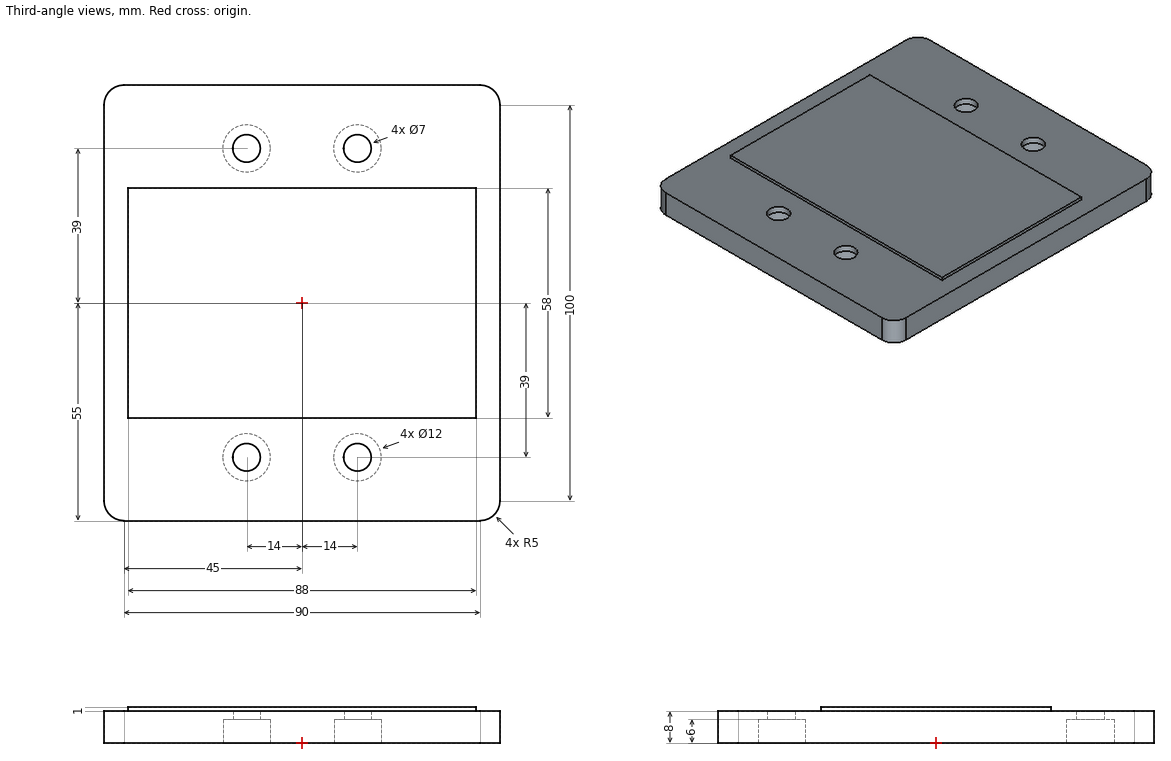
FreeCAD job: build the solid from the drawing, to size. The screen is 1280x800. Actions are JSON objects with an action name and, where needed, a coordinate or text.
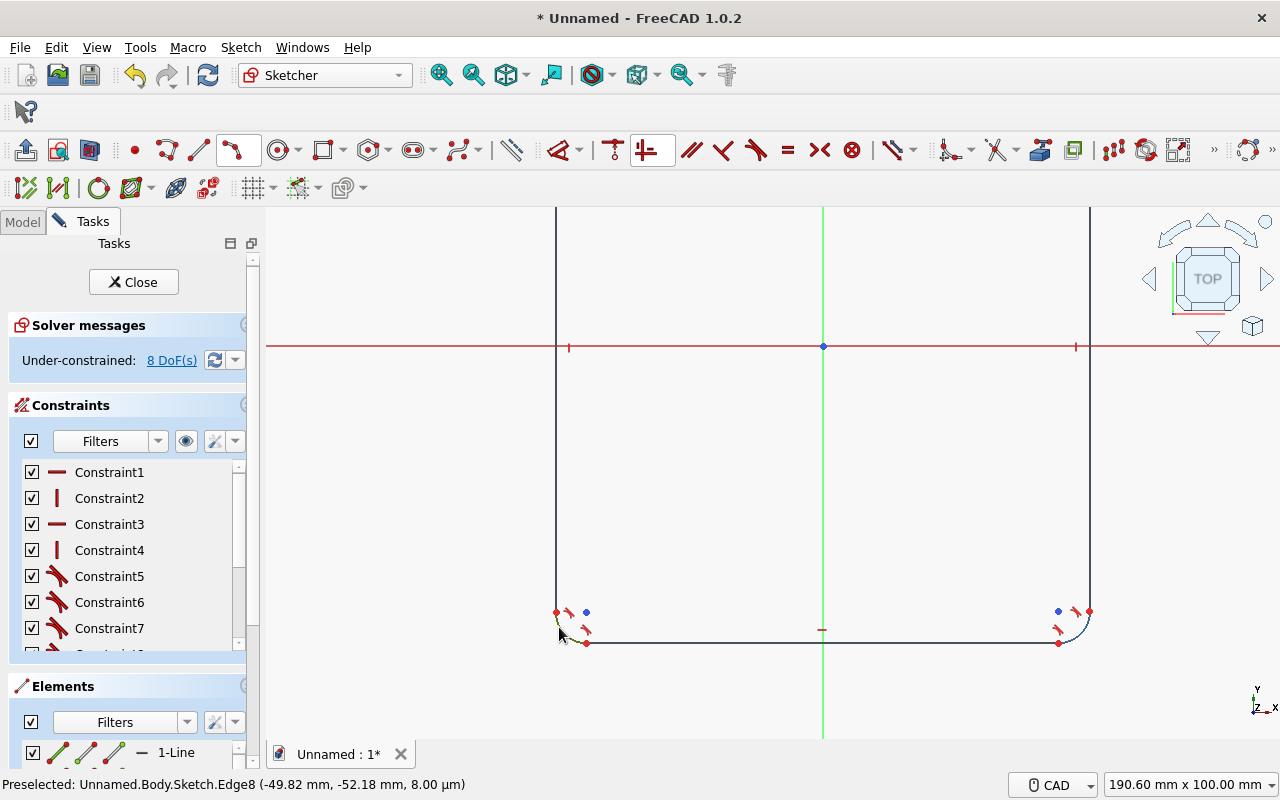
{"action": "left_click", "coordinate": [788, 150]}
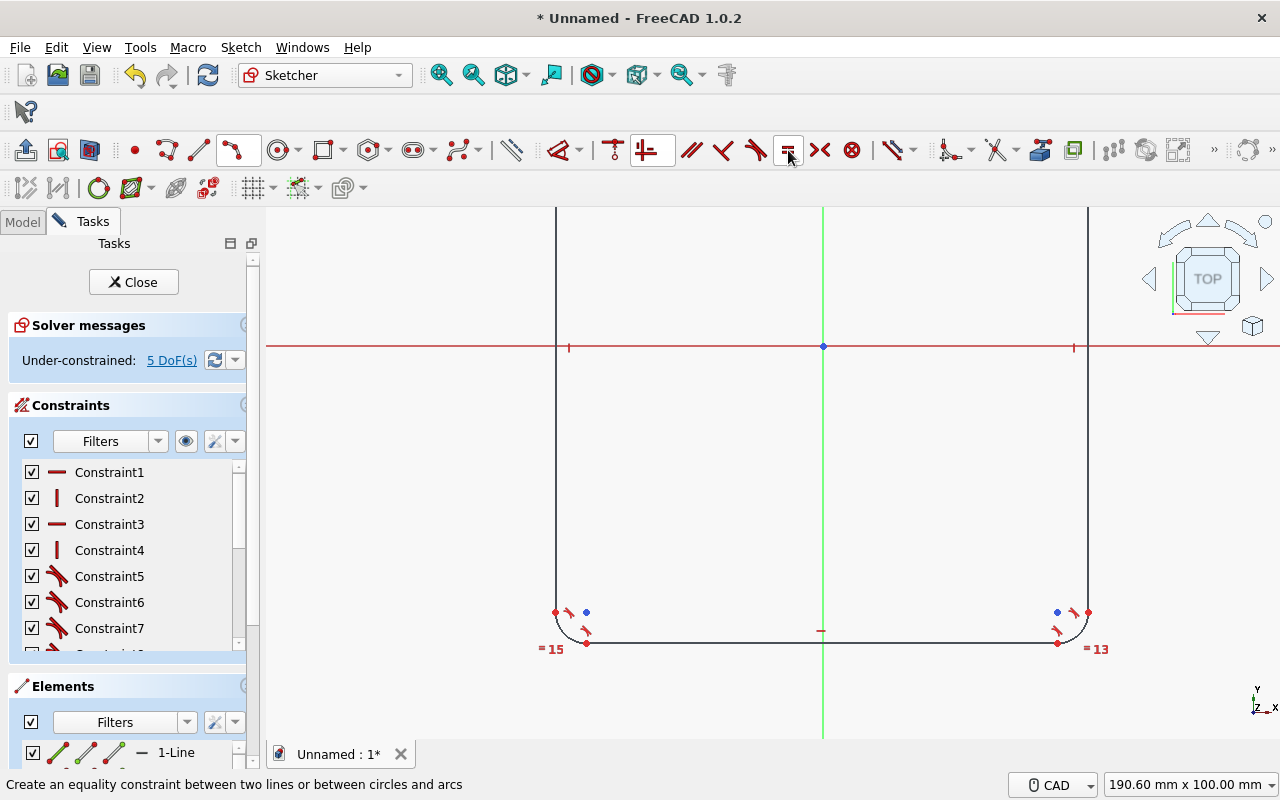
{"action": "key", "text": "d"}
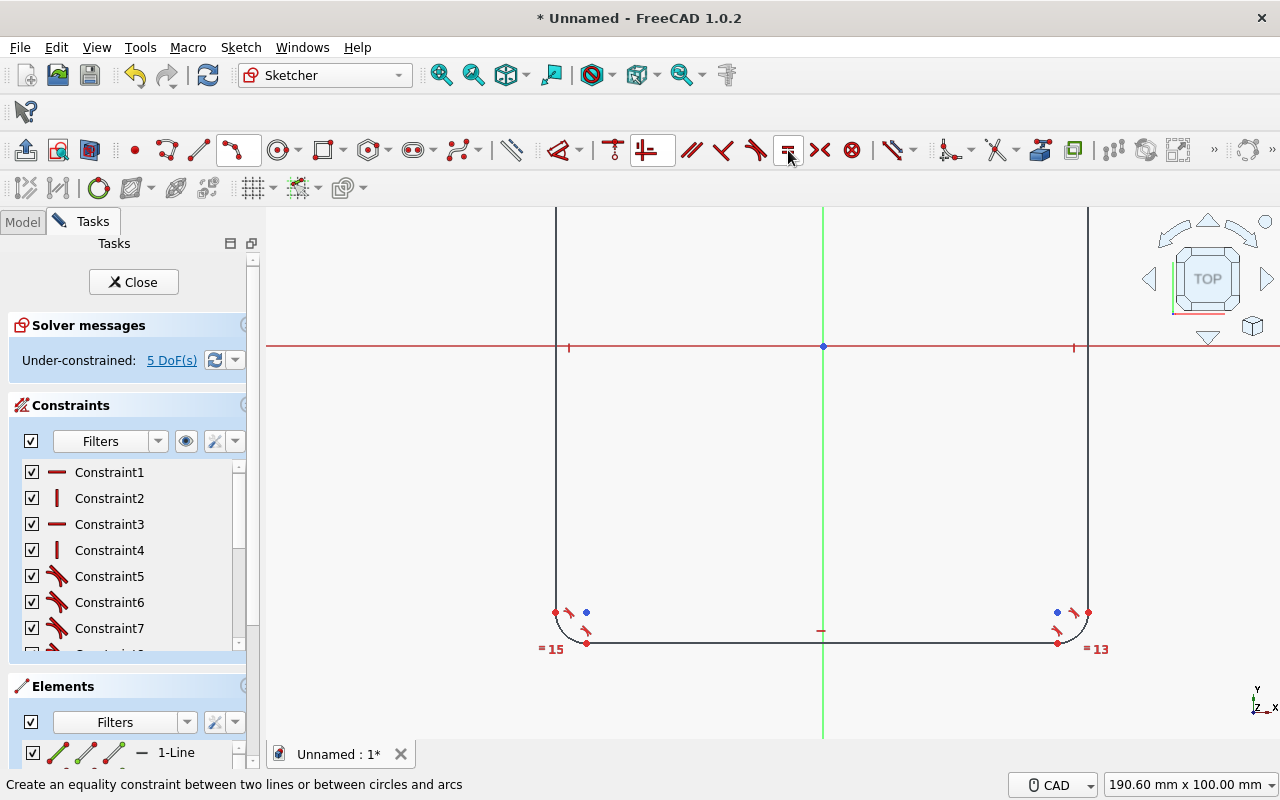
{"action": "scroll", "coordinate": [1071, 640], "scroll_direction": "up", "scroll_amount": 3}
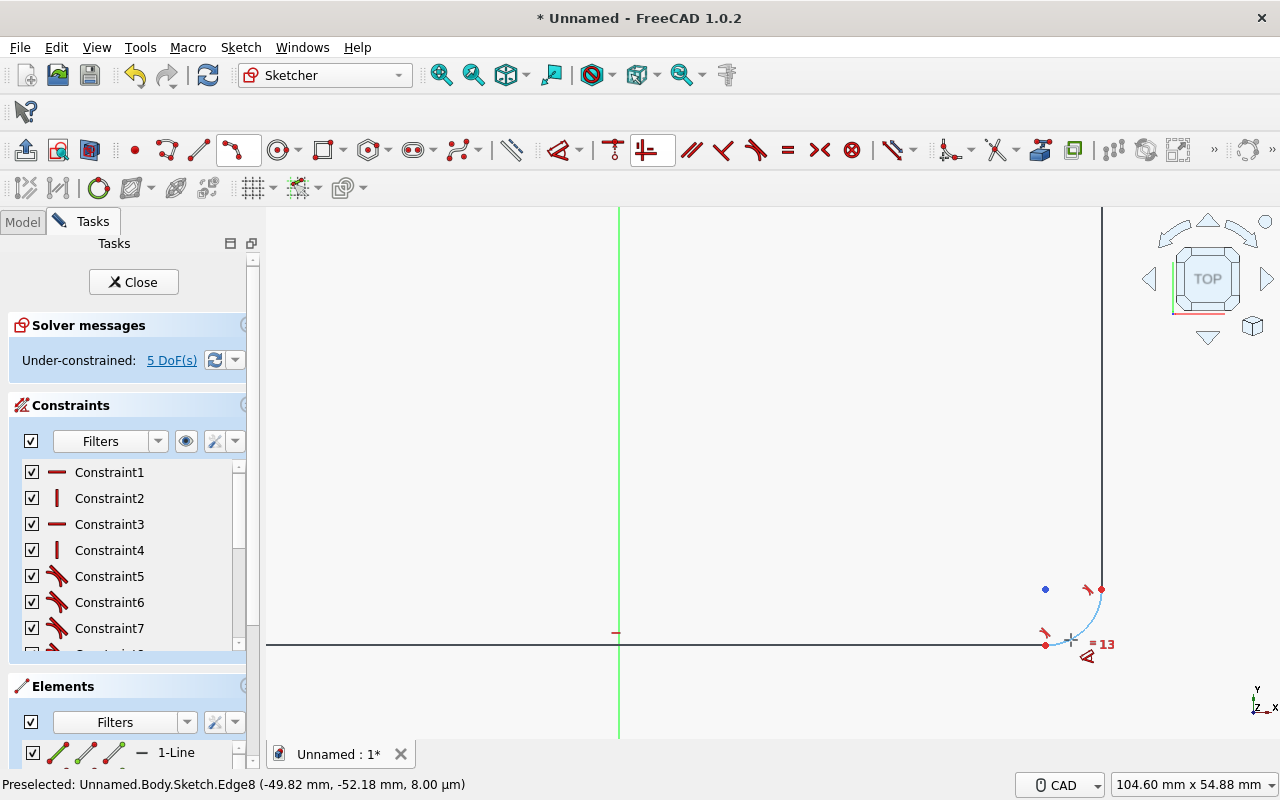
{"action": "left_click", "coordinate": [1071, 639]}
{"action": "left_click", "coordinate": [1086, 667]}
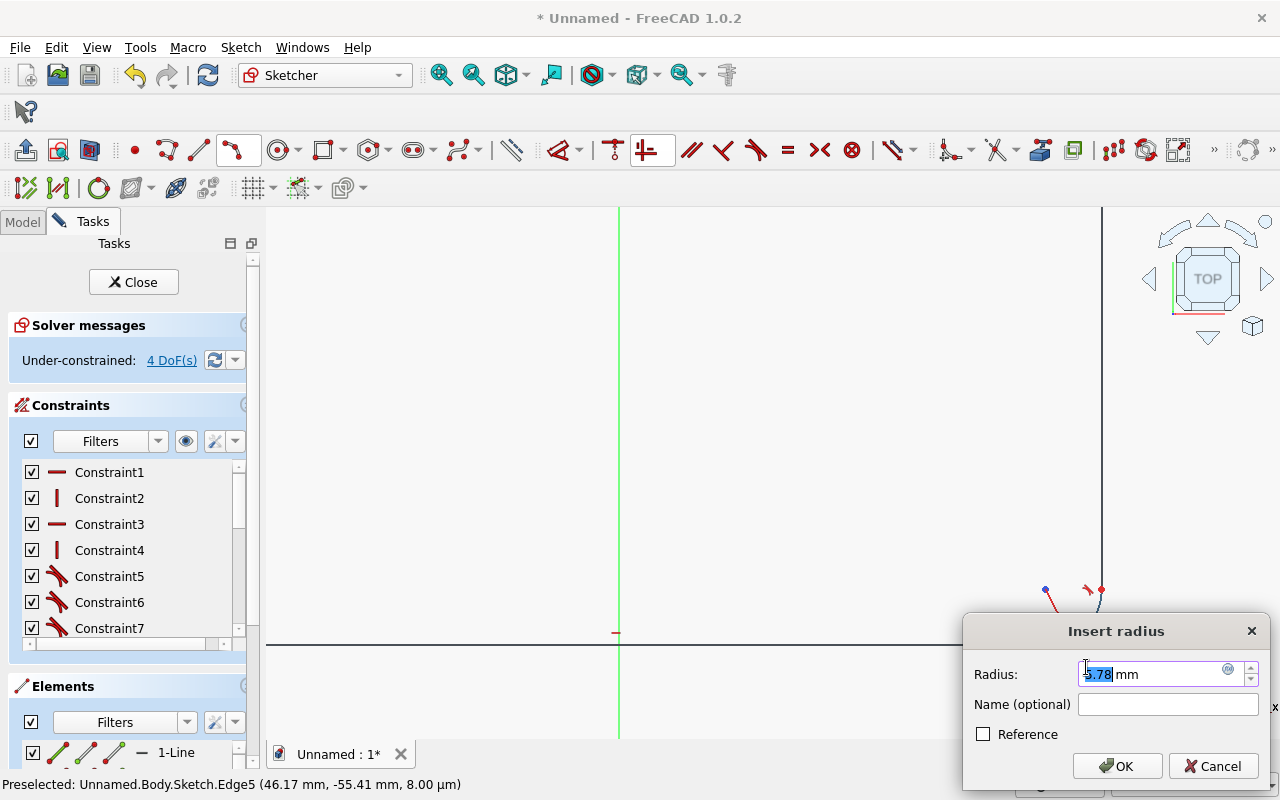
{"action": "type", "text": "5"}
{"action": "key", "text": "Return"}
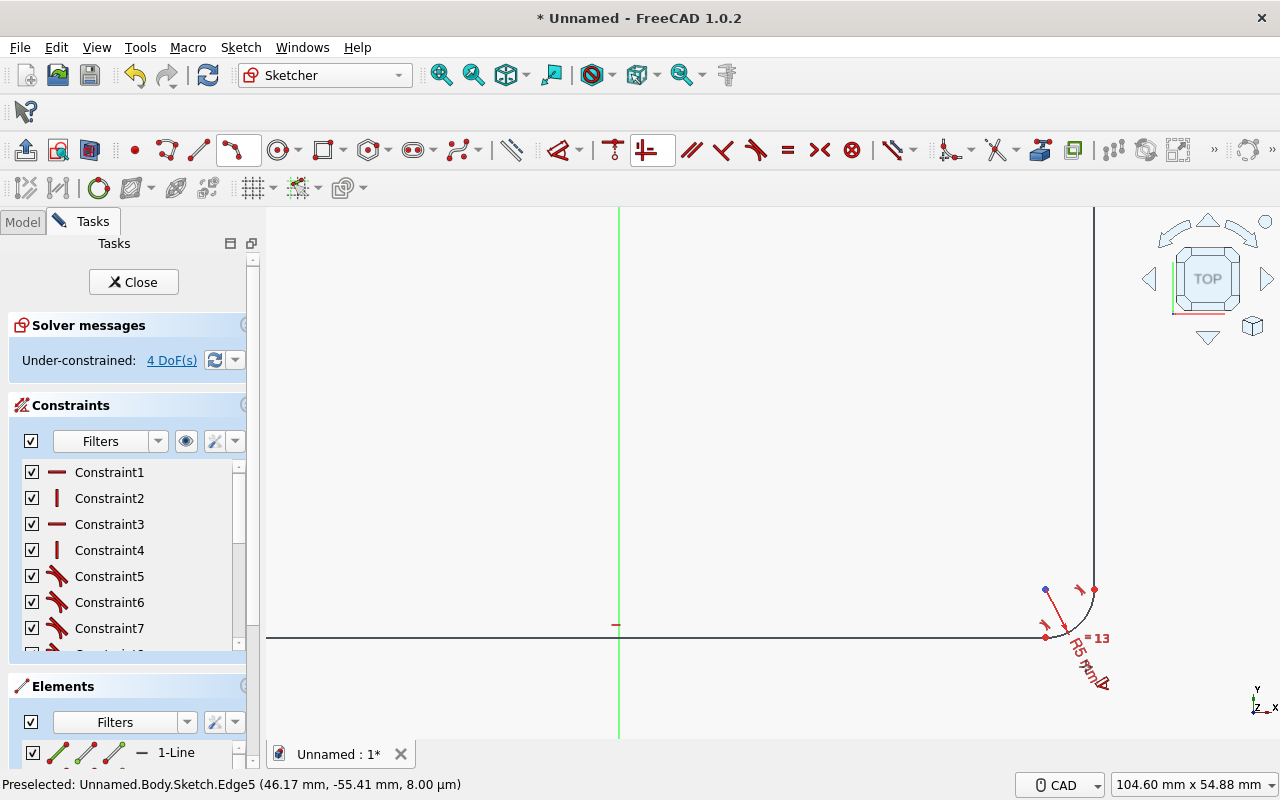
{"action": "left_click", "coordinate": [445, 638]}
{"action": "left_click", "coordinate": [670, 672]}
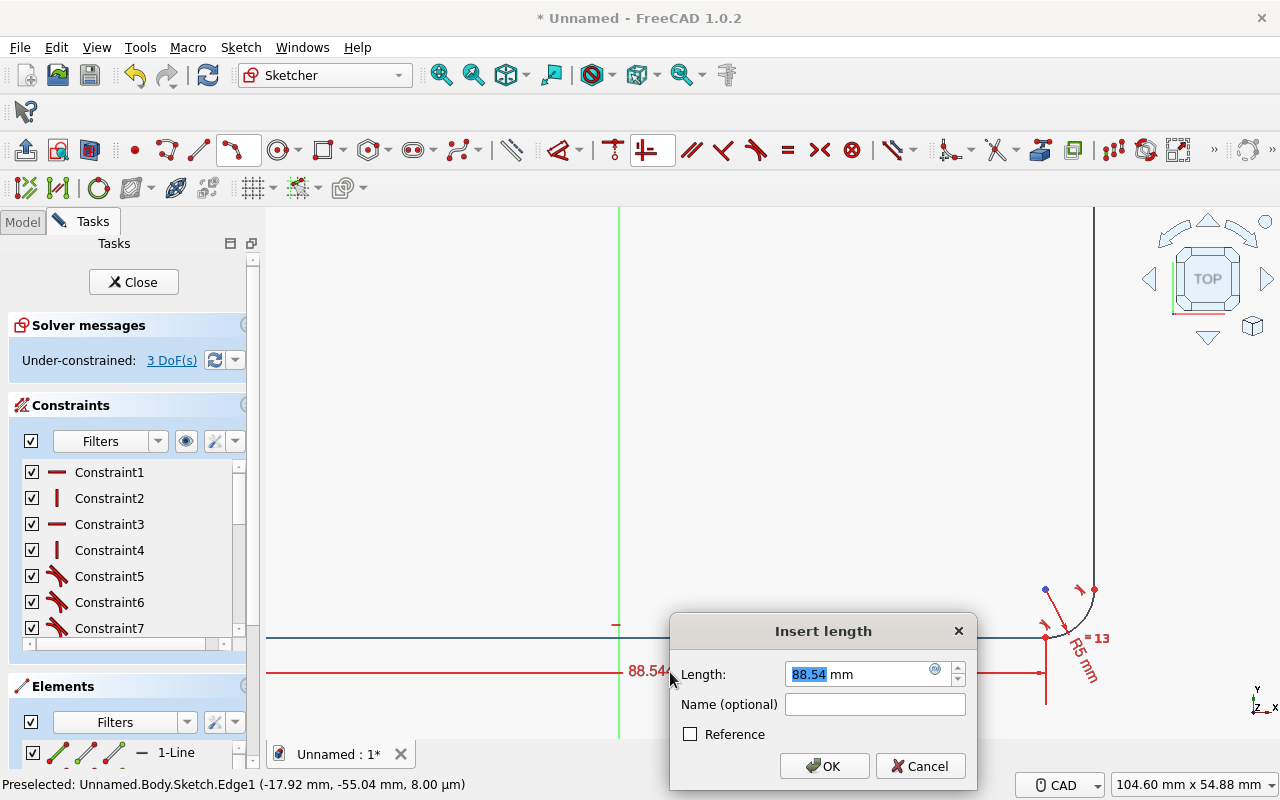
{"action": "type", "text": "90"}
{"action": "key", "text": "Return"}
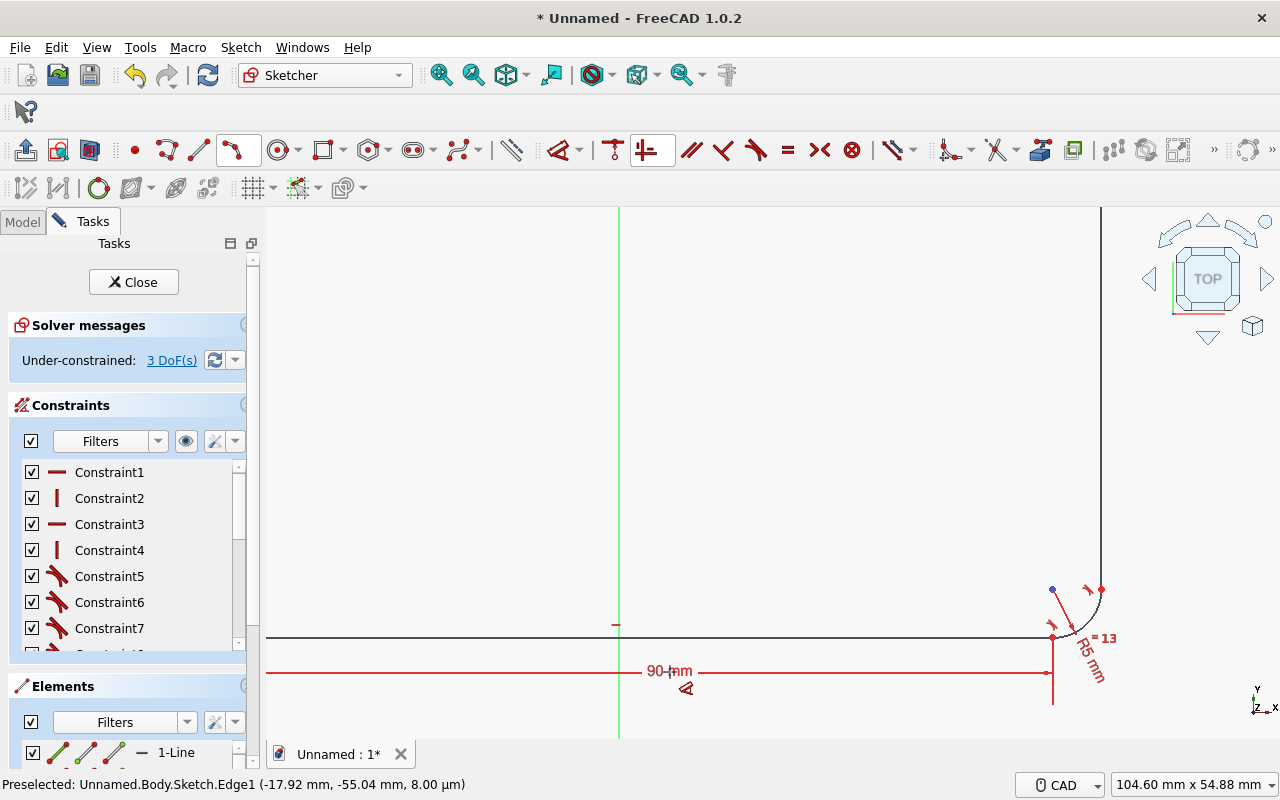
{"action": "left_click", "coordinate": [1101, 299]}
{"action": "left_click", "coordinate": [1067, 412]}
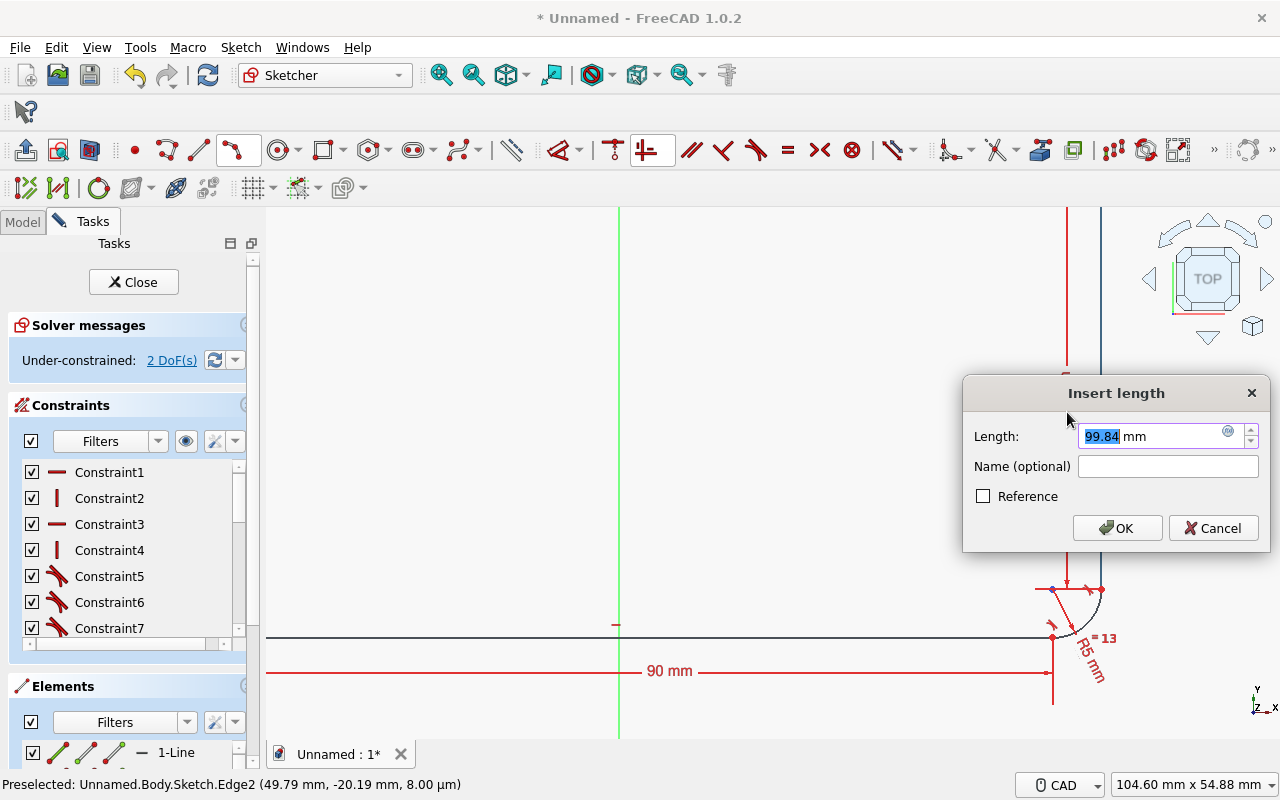
{"action": "type", "text": "100"}
{"action": "key", "text": "Return"}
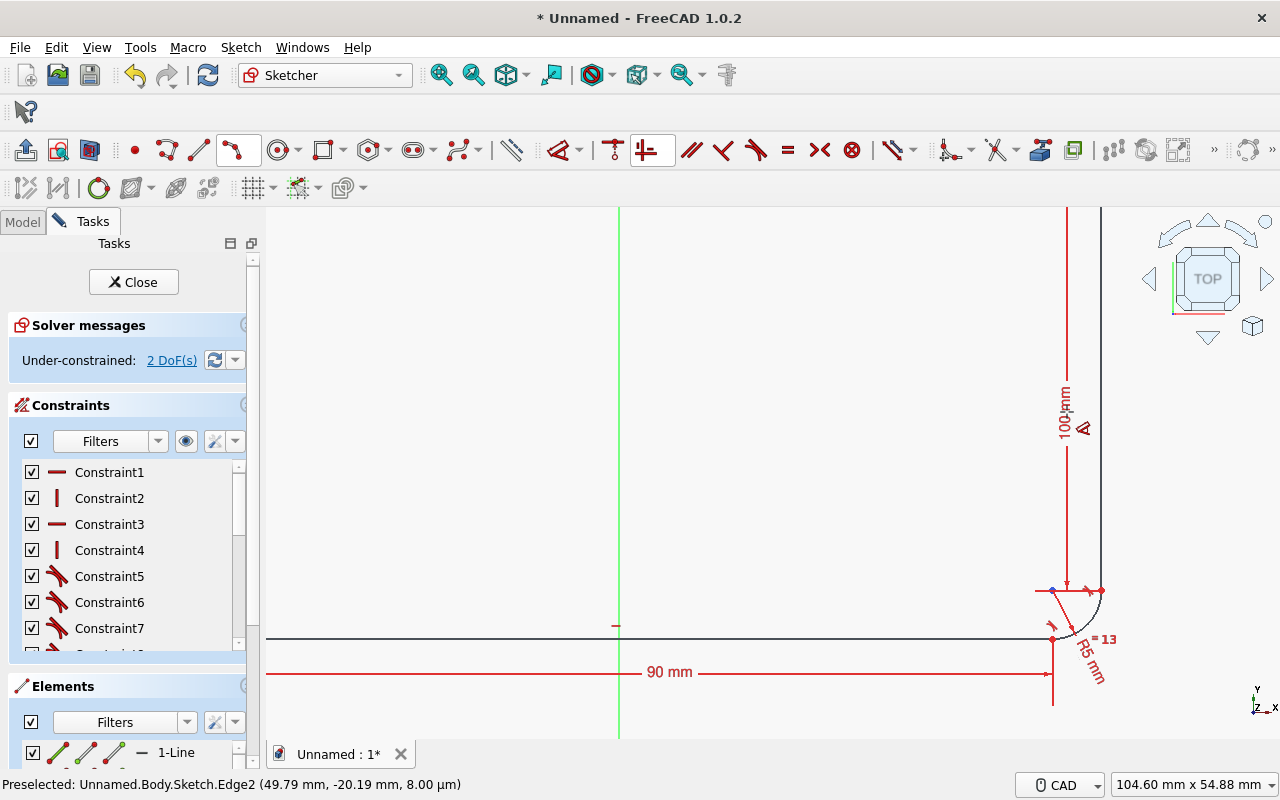
{"action": "scroll", "coordinate": [741, 632], "scroll_direction": "down", "scroll_amount": 6}